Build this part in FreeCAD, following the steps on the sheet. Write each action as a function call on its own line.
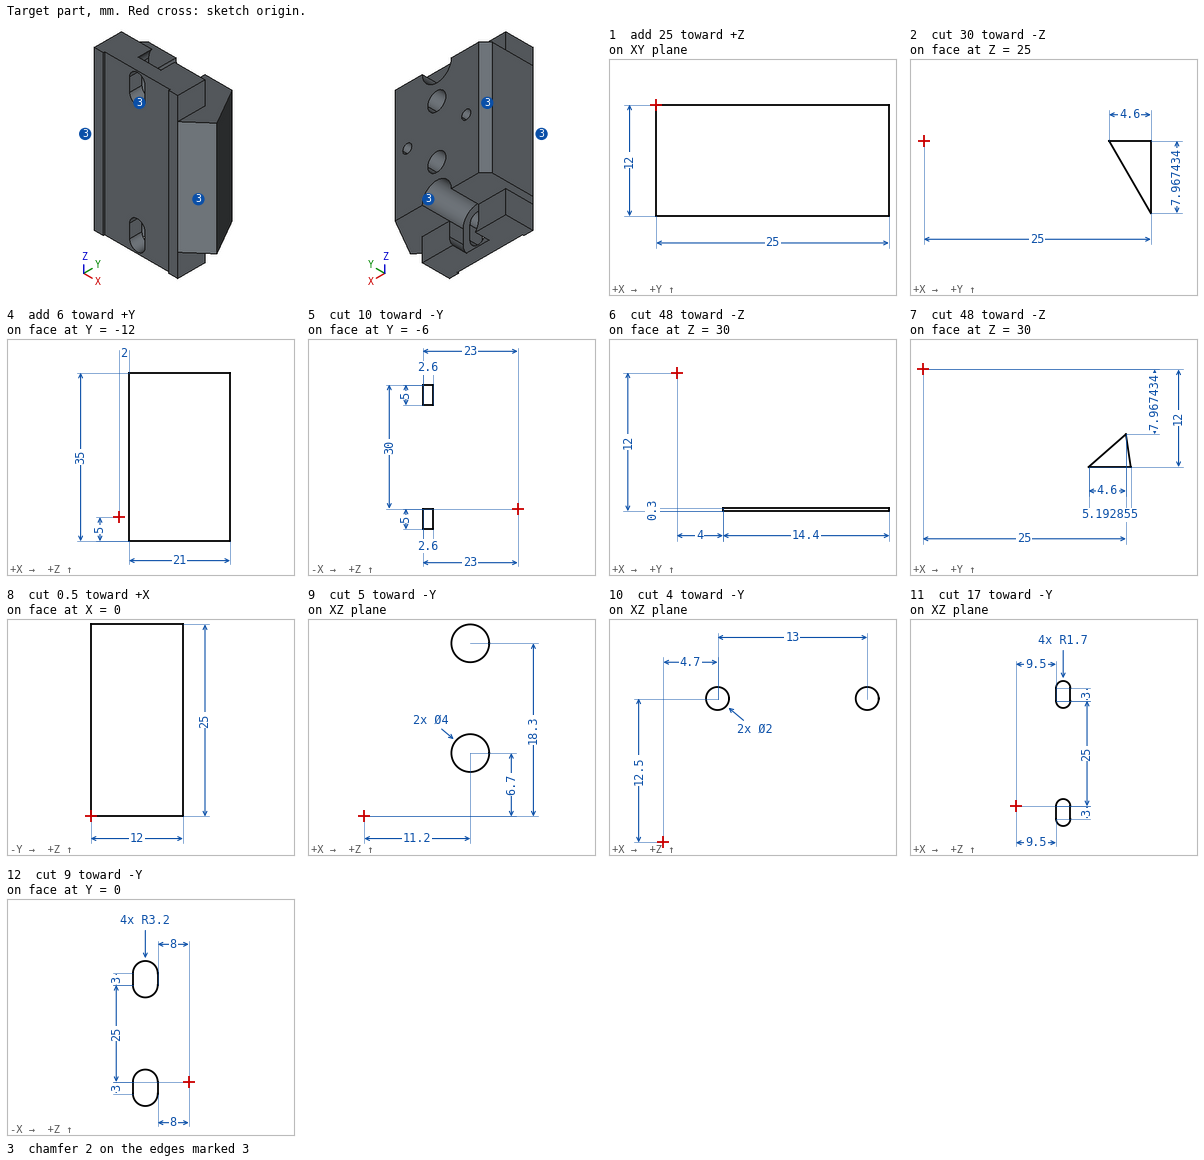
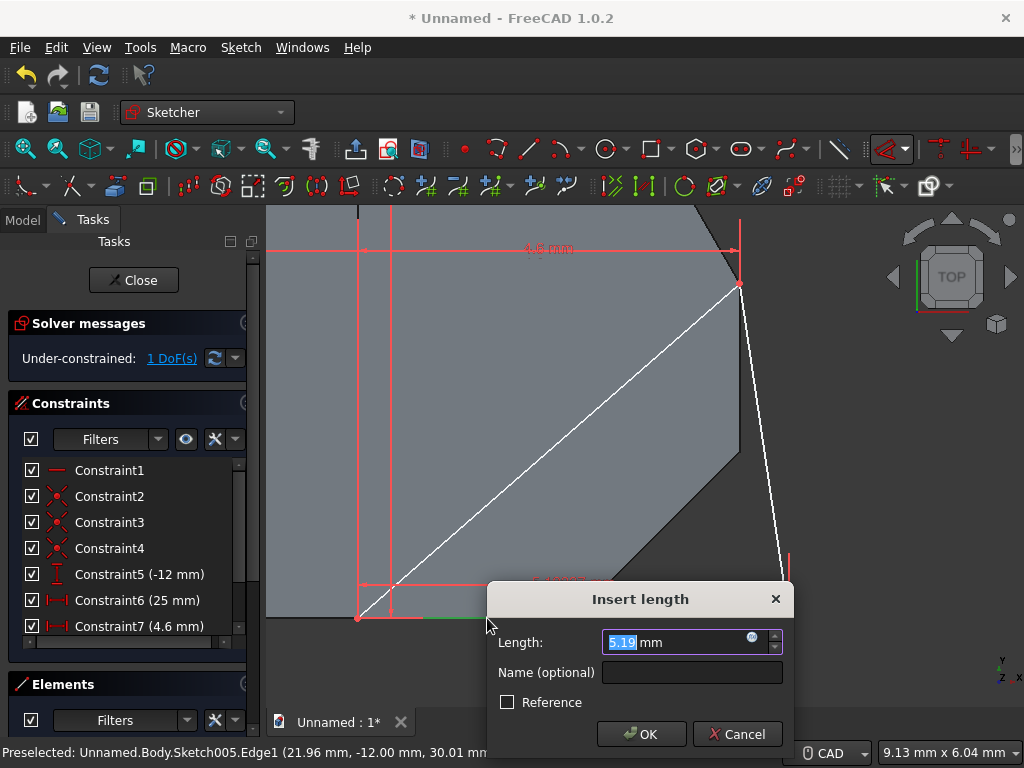
text(5.192855)
key(Return)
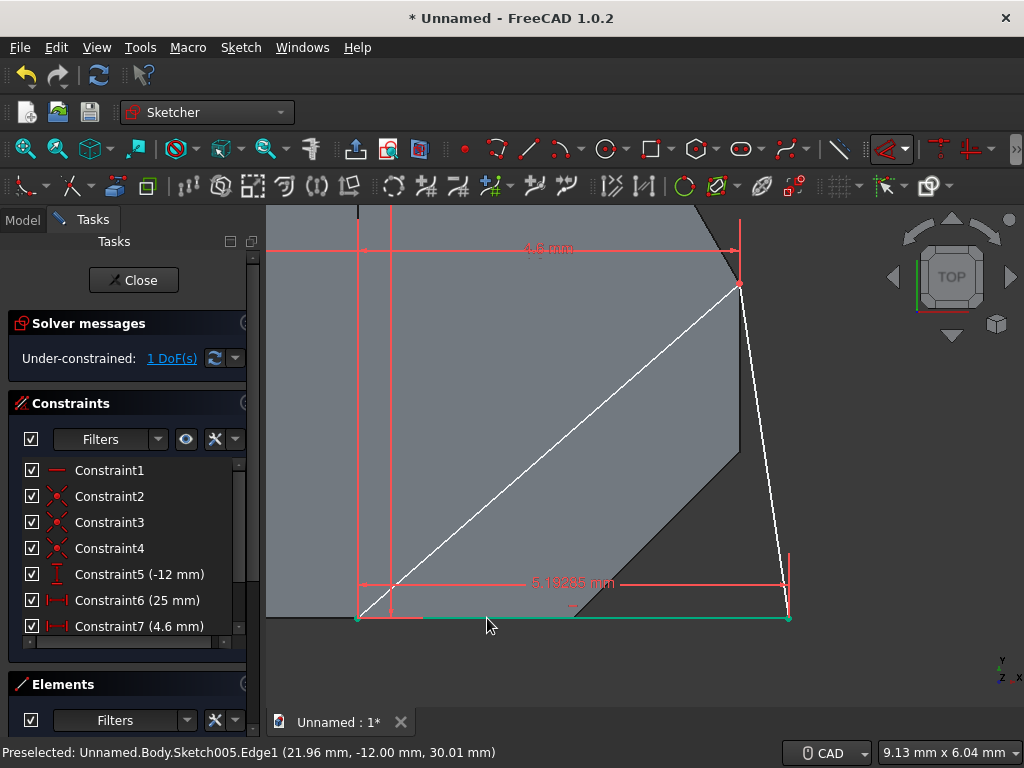
click(740, 284)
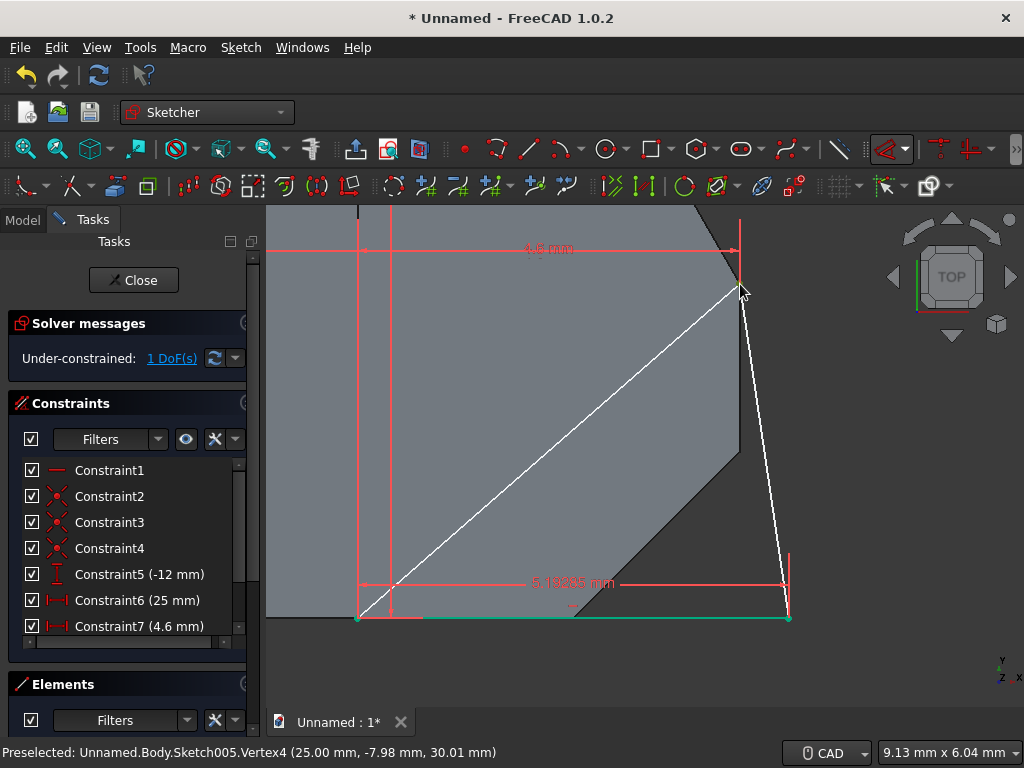
key(i)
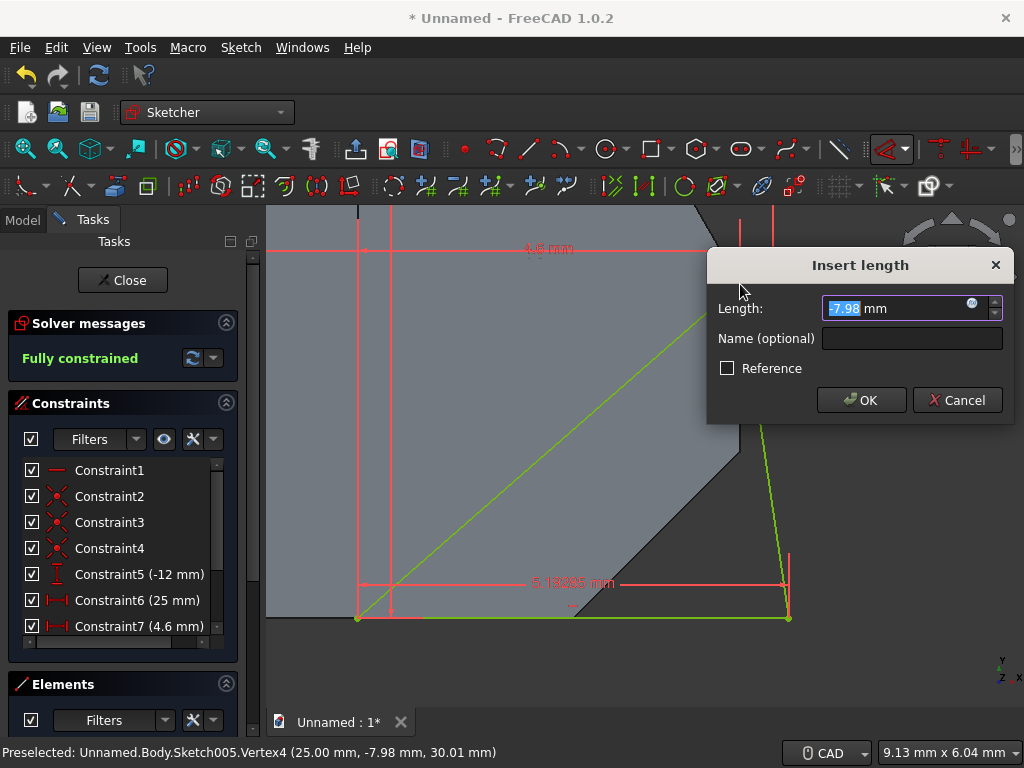
text(-7.967434)
key(Return)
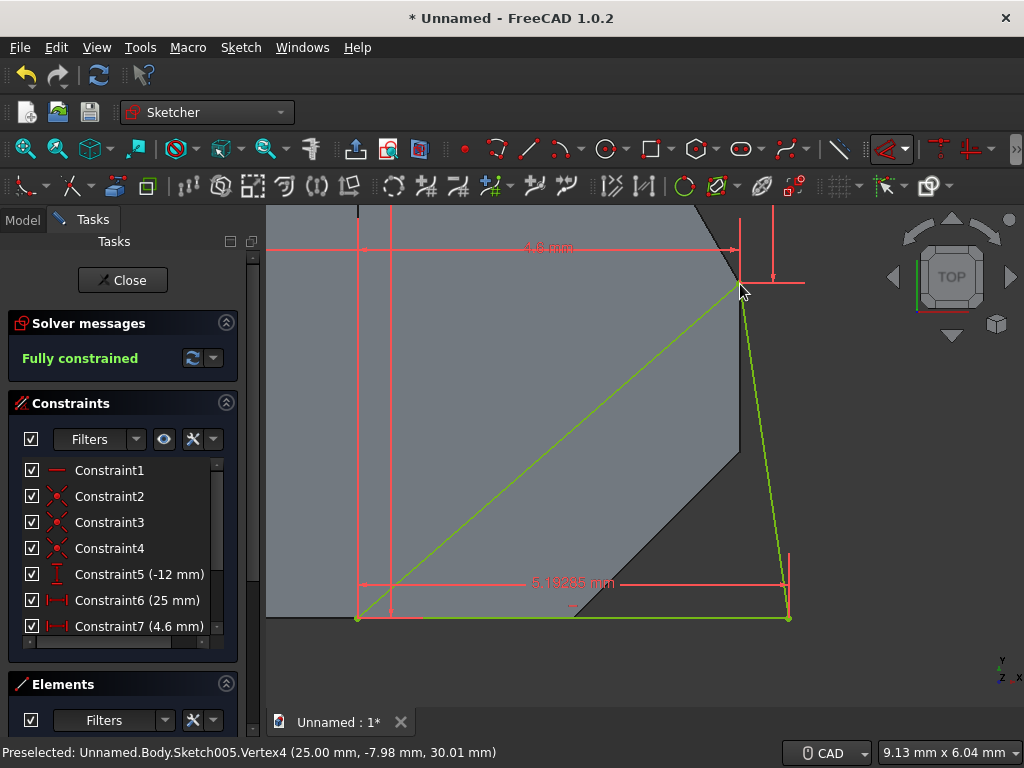
click(123, 280)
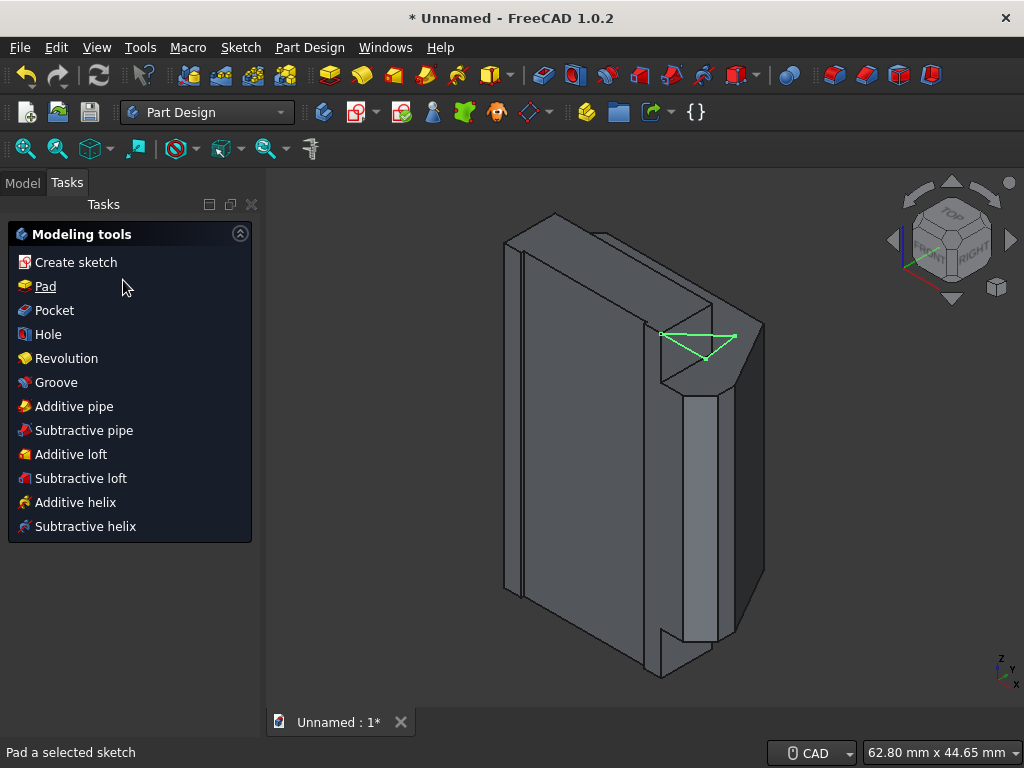
click(544, 76)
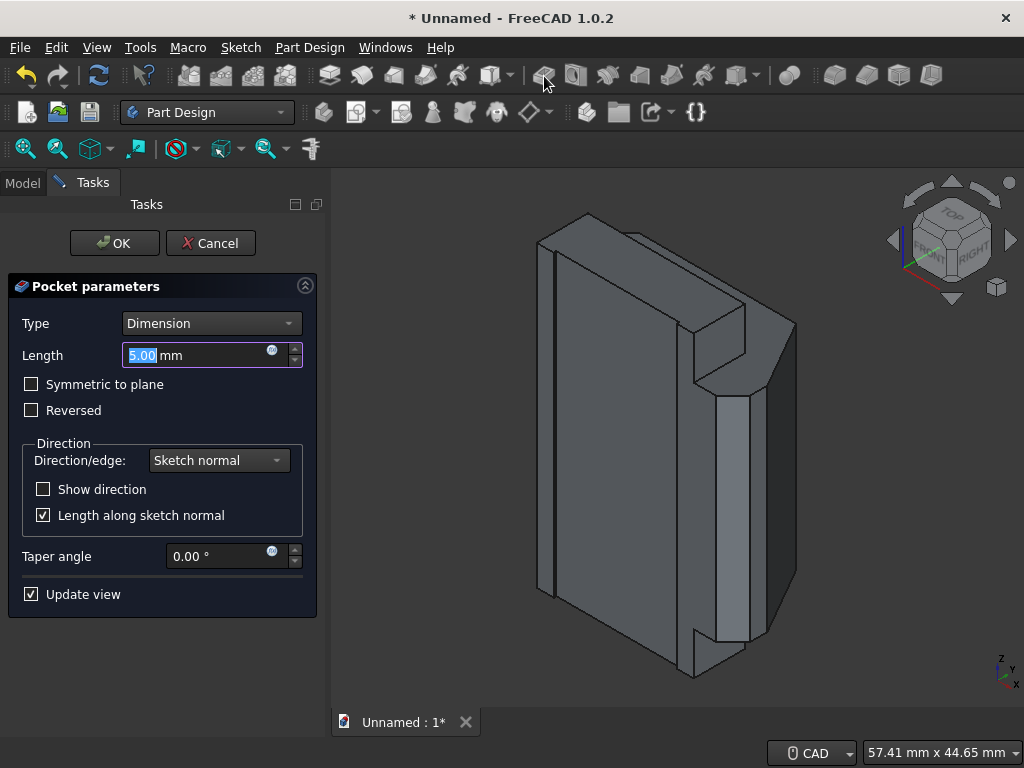
text(48)
key(Tab)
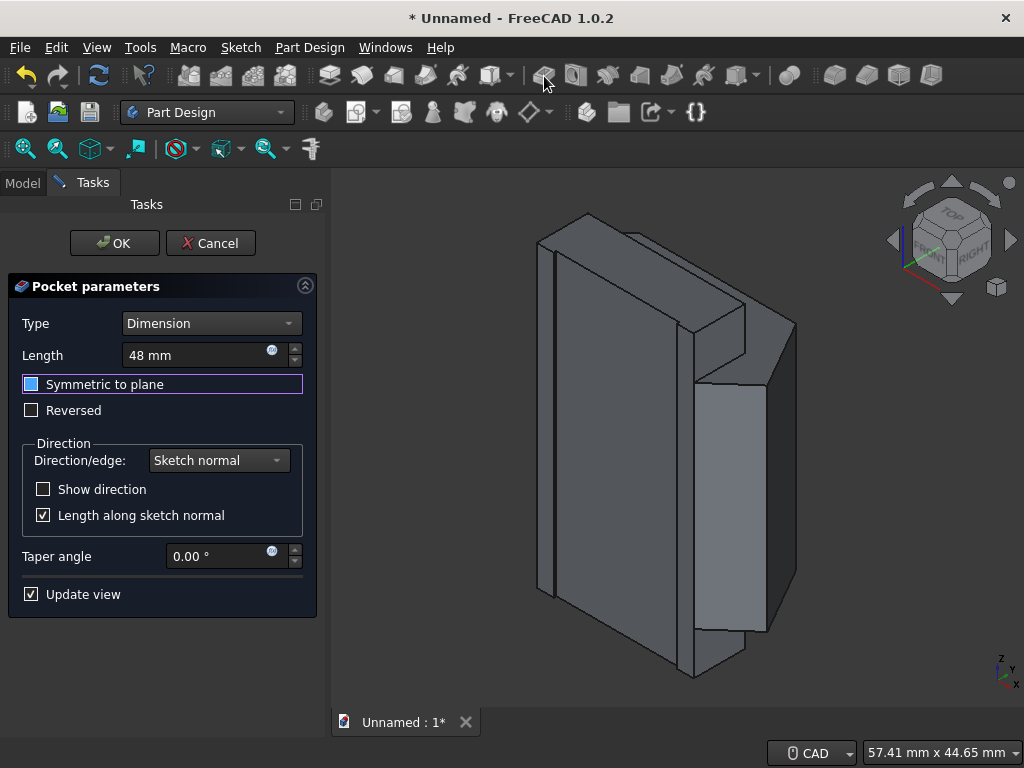
click(115, 243)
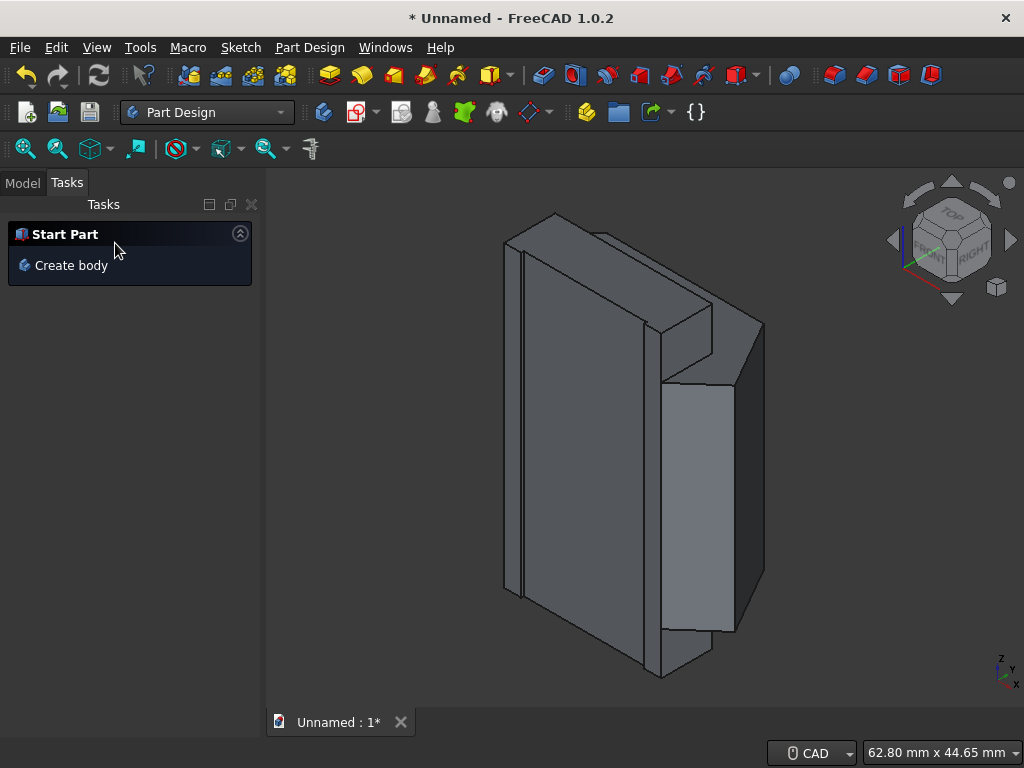
key(6)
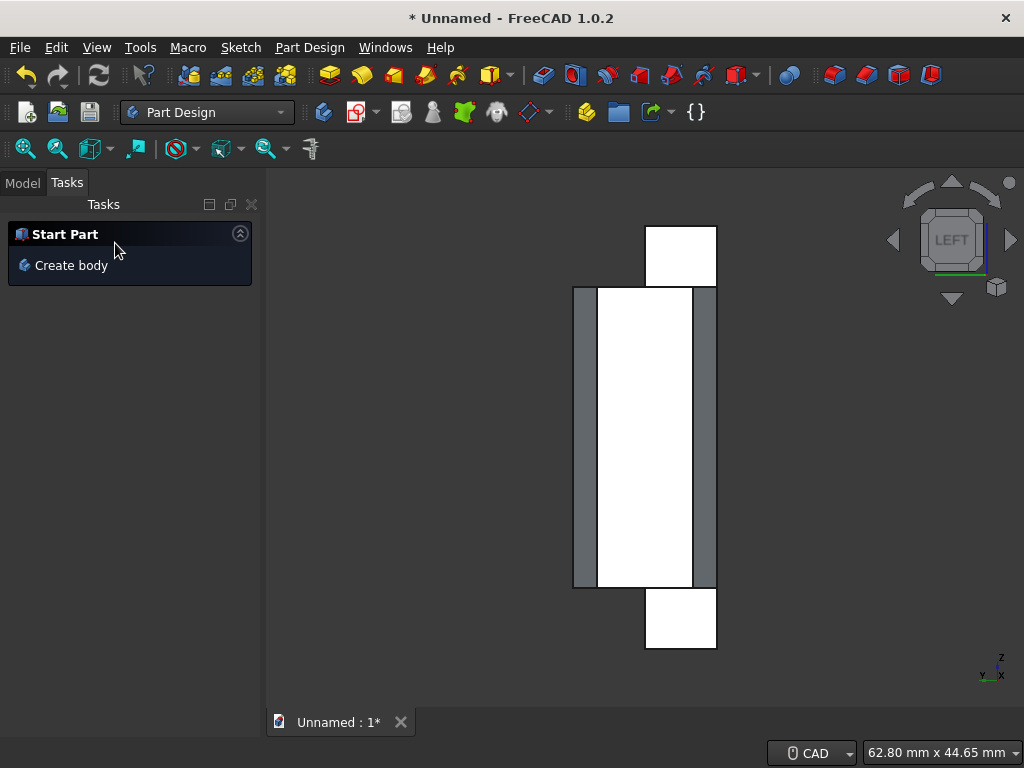
click(645, 350)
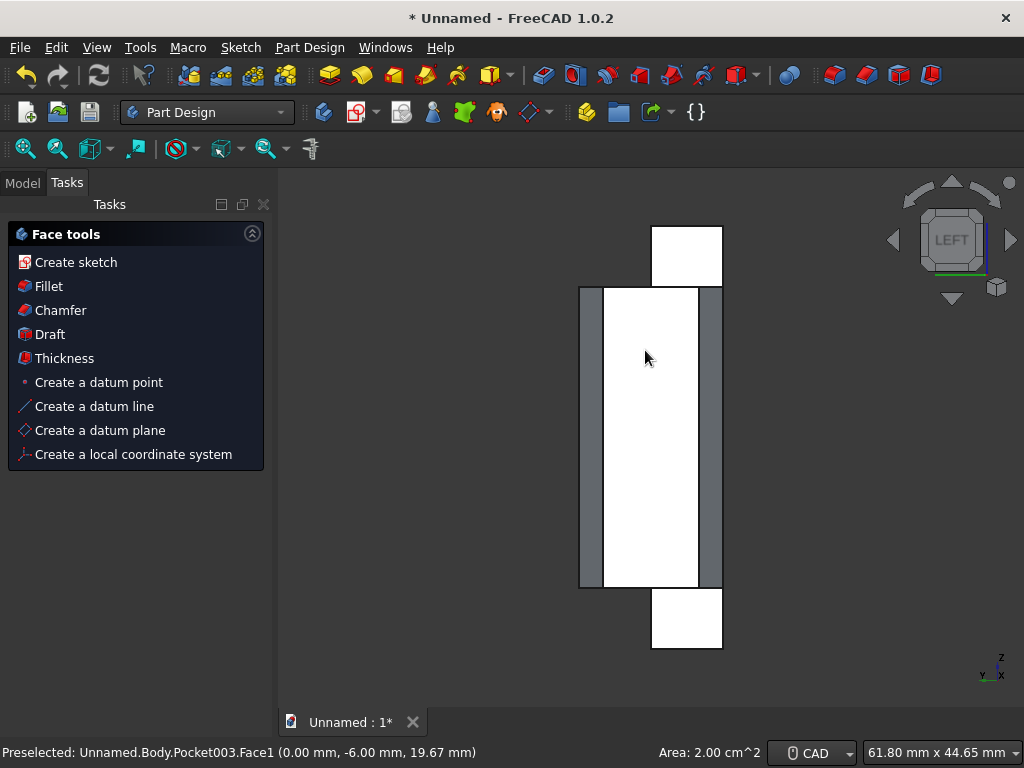
click(356, 112)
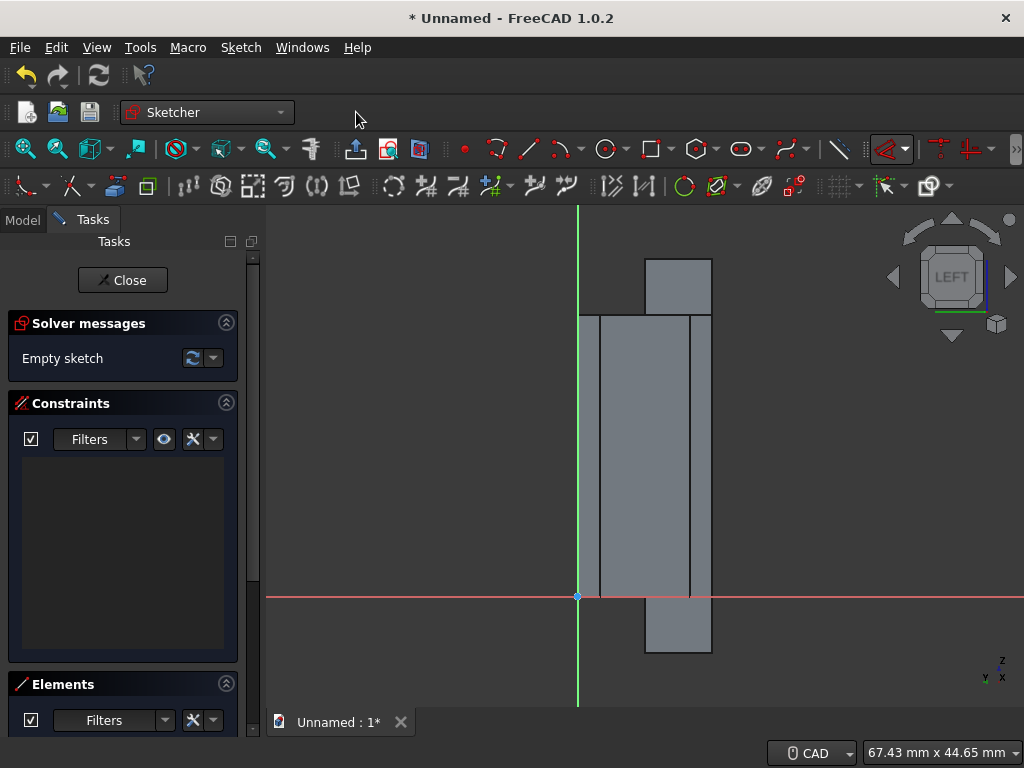
click(652, 150)